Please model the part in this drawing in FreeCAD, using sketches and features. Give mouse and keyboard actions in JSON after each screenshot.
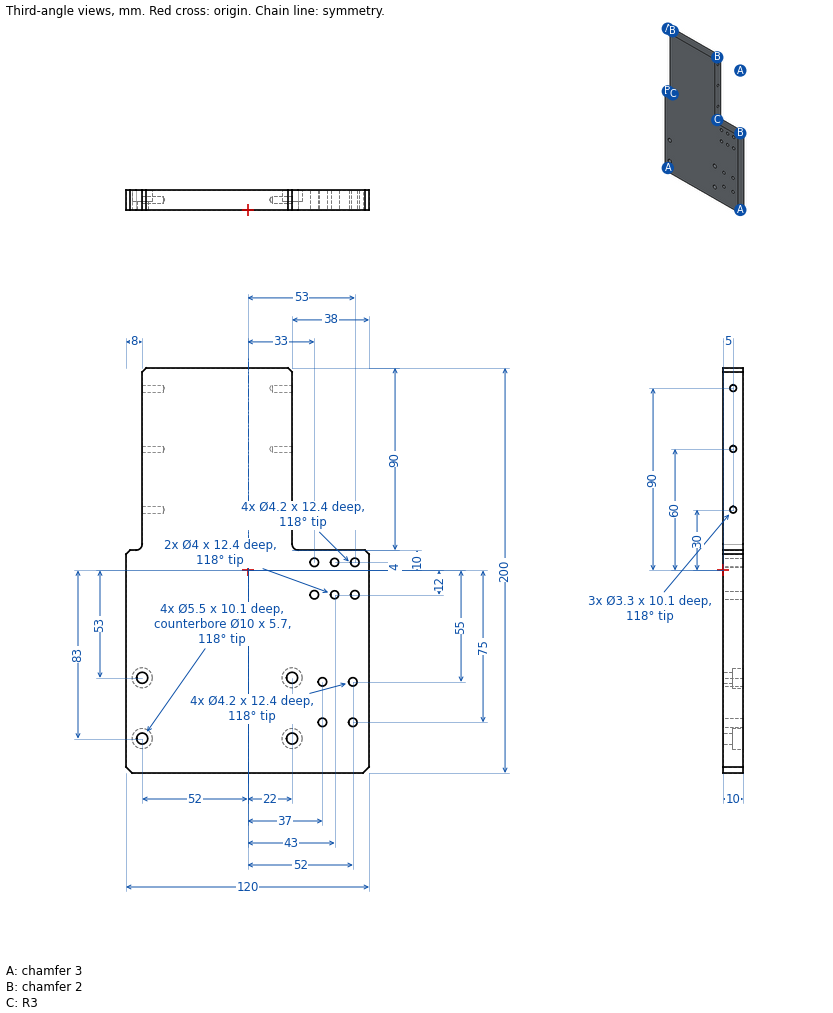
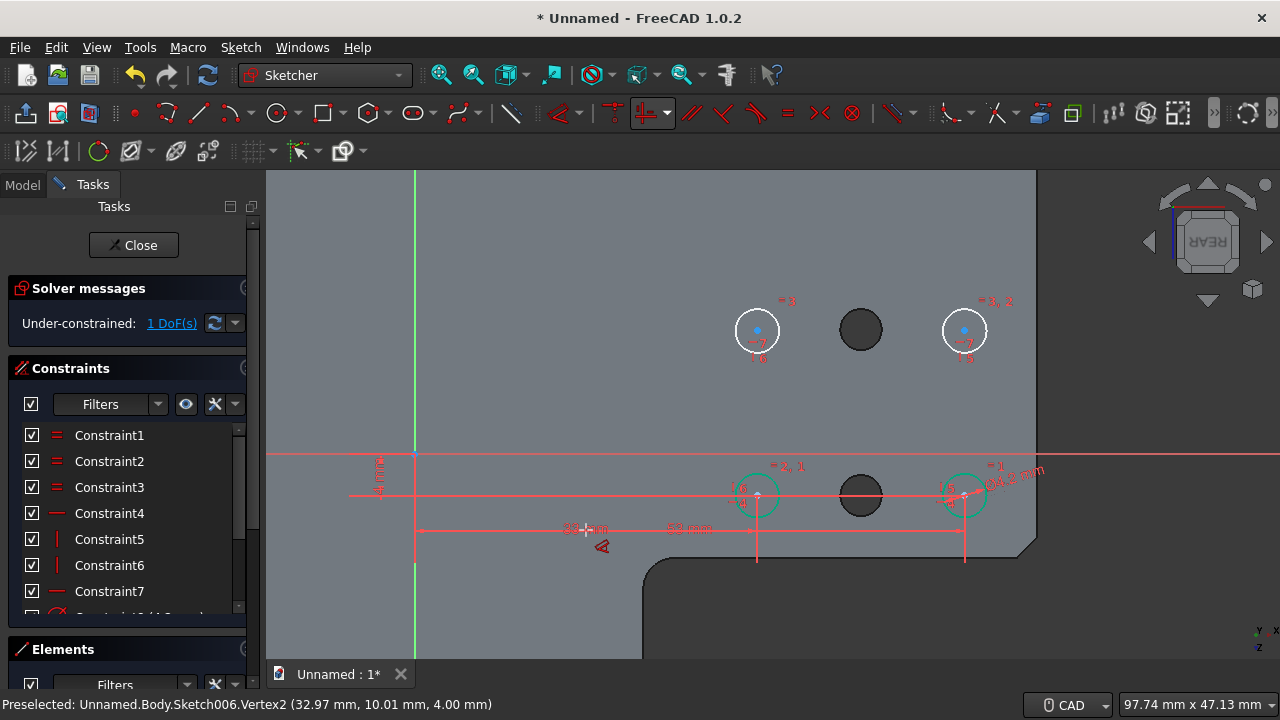
{"action": "left_click", "coordinate": [965, 331]}
{"action": "left_click", "coordinate": [381, 393]}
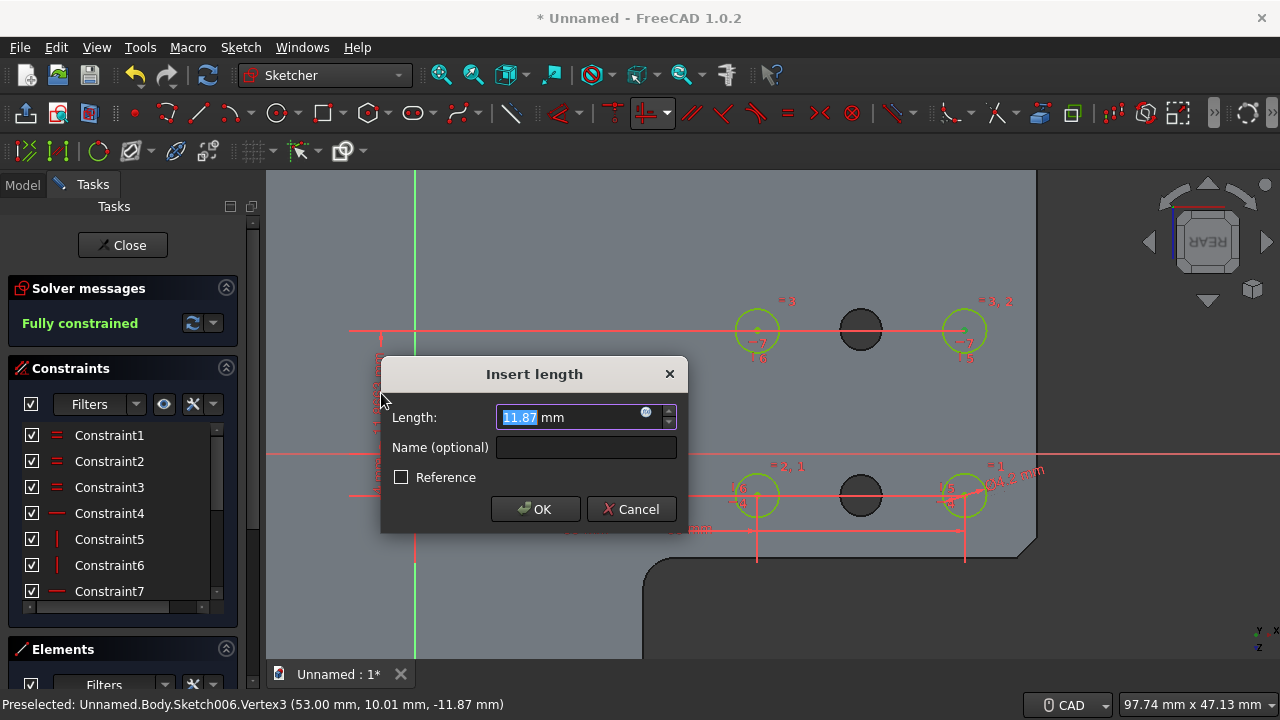
{"action": "type", "text": "12"}
{"action": "key", "text": "Return"}
{"action": "key", "text": "Escape"}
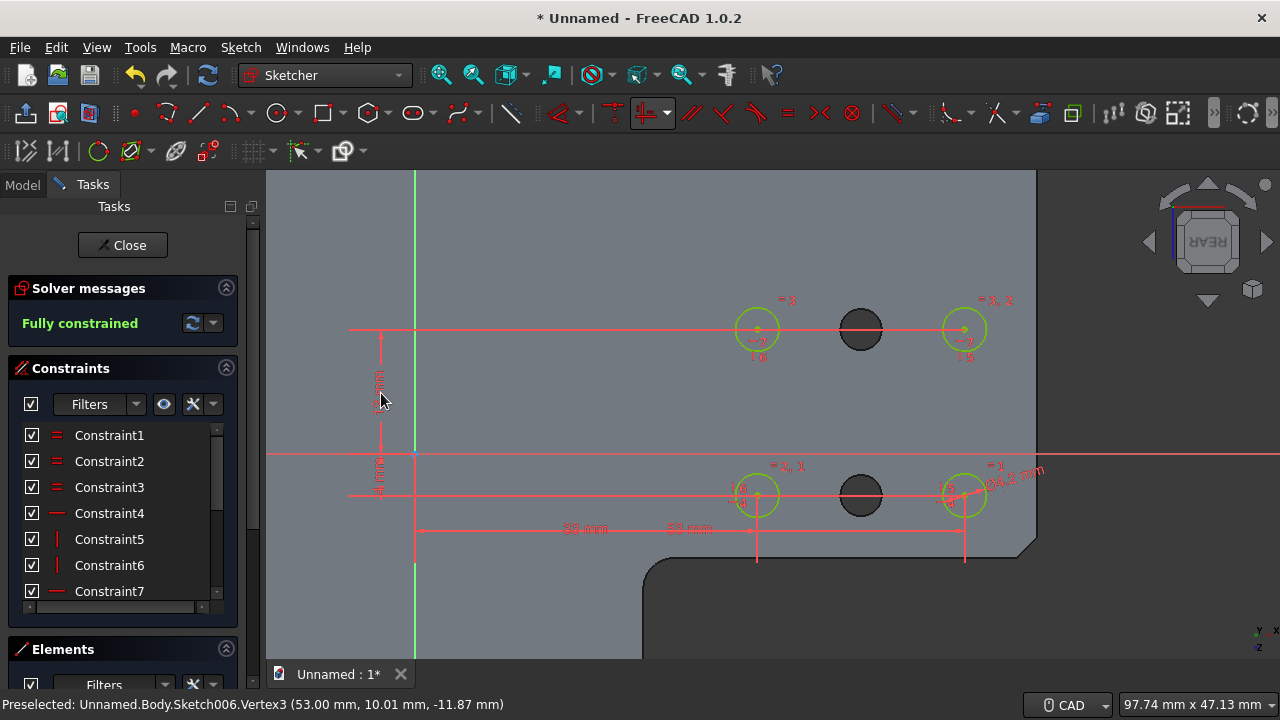
{"action": "left_click", "coordinate": [123, 245]}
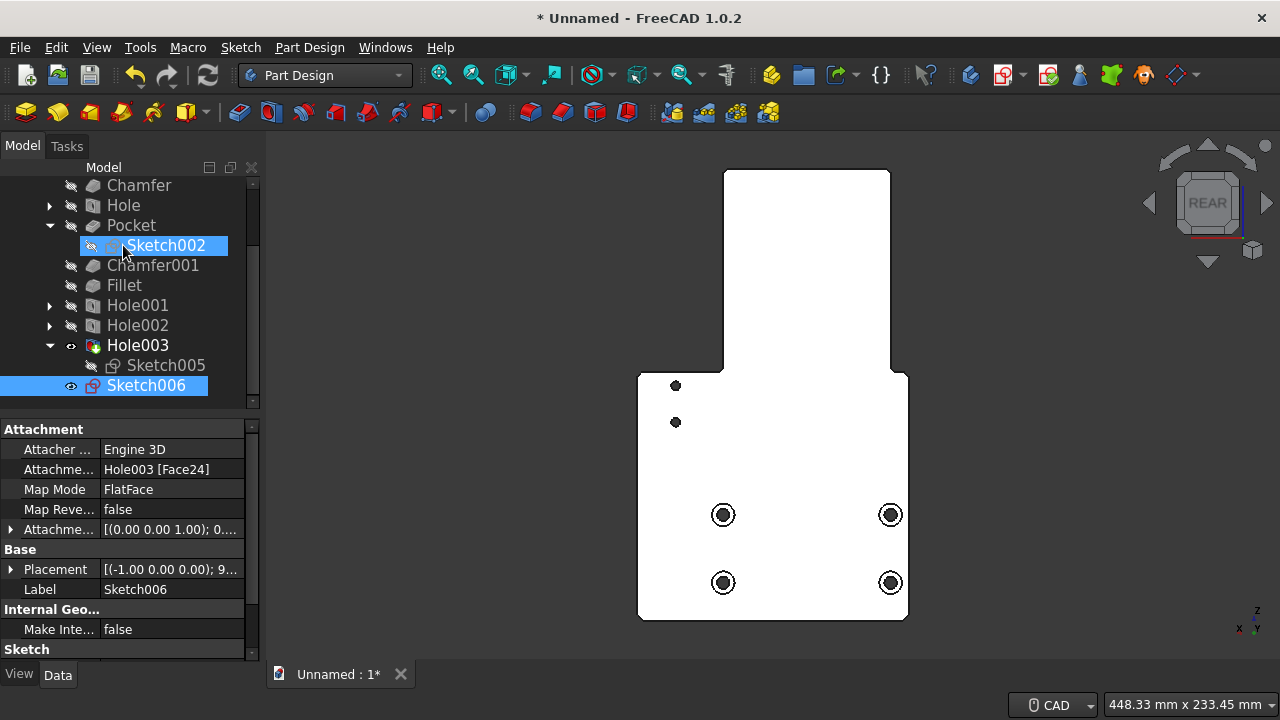
{"action": "left_click", "coordinate": [272, 112]}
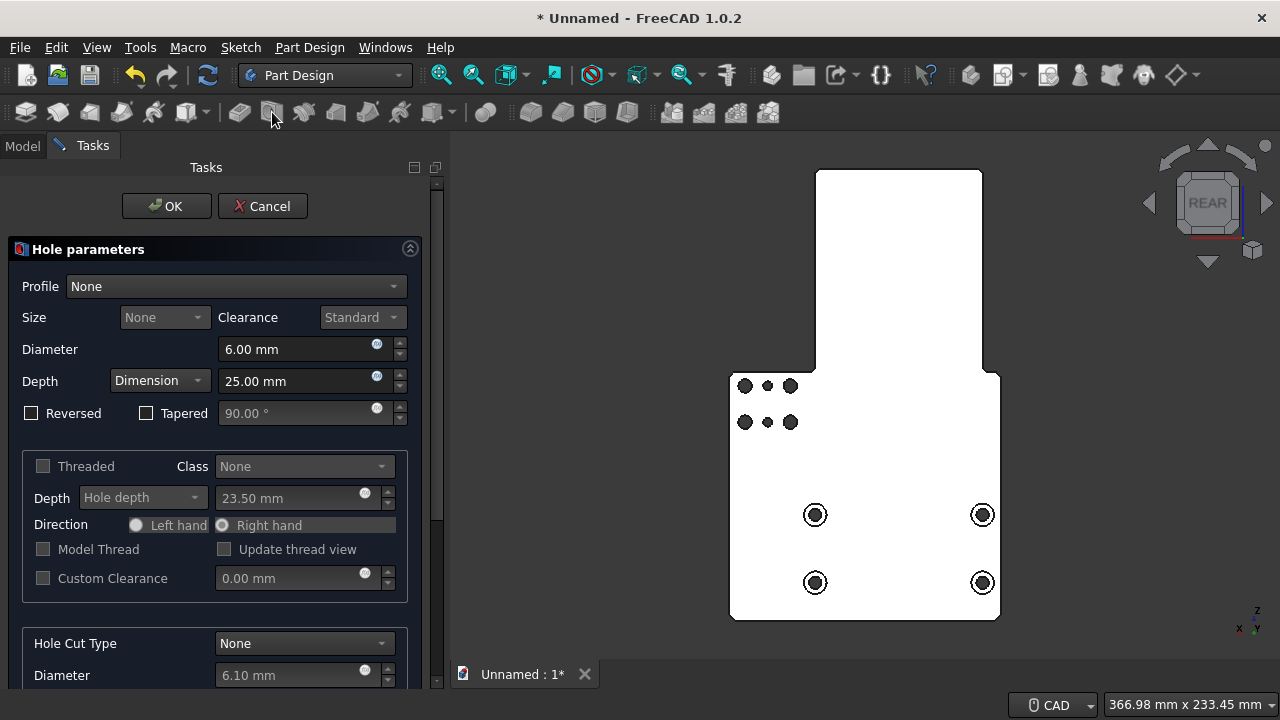
{"action": "triple_click", "coordinate": [305, 349]}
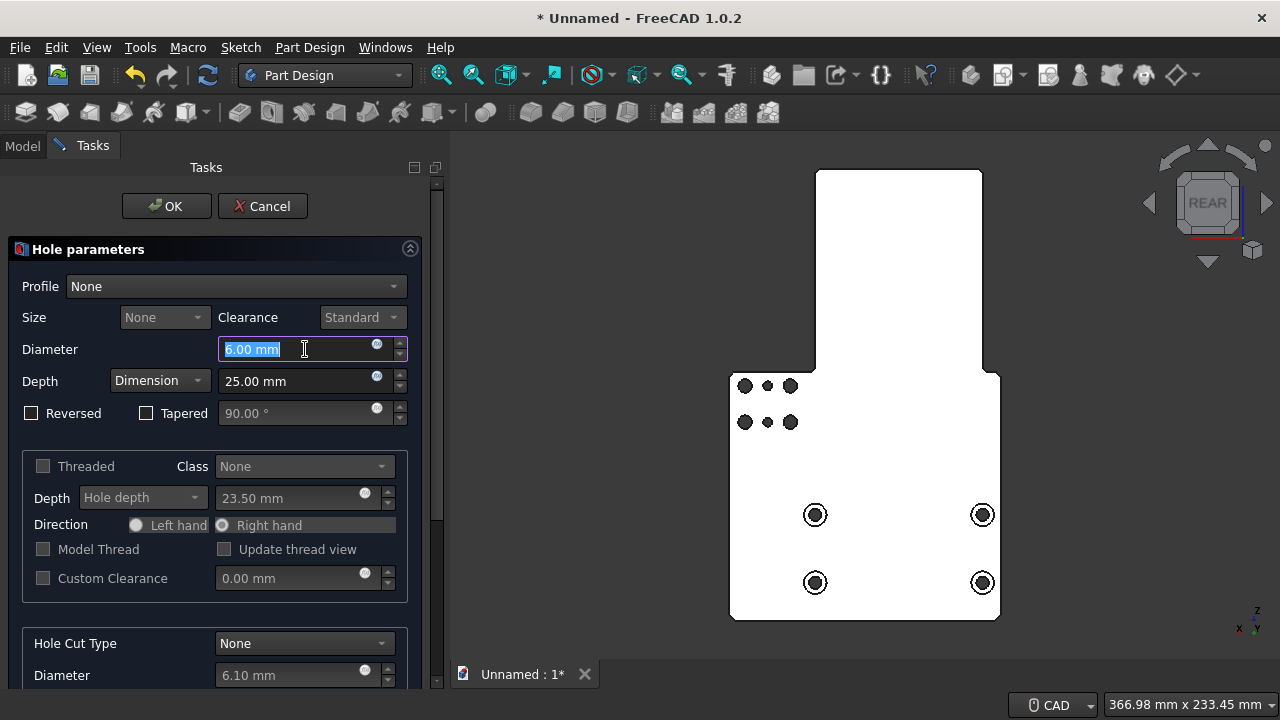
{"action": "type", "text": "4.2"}
{"action": "key", "text": "Tab"}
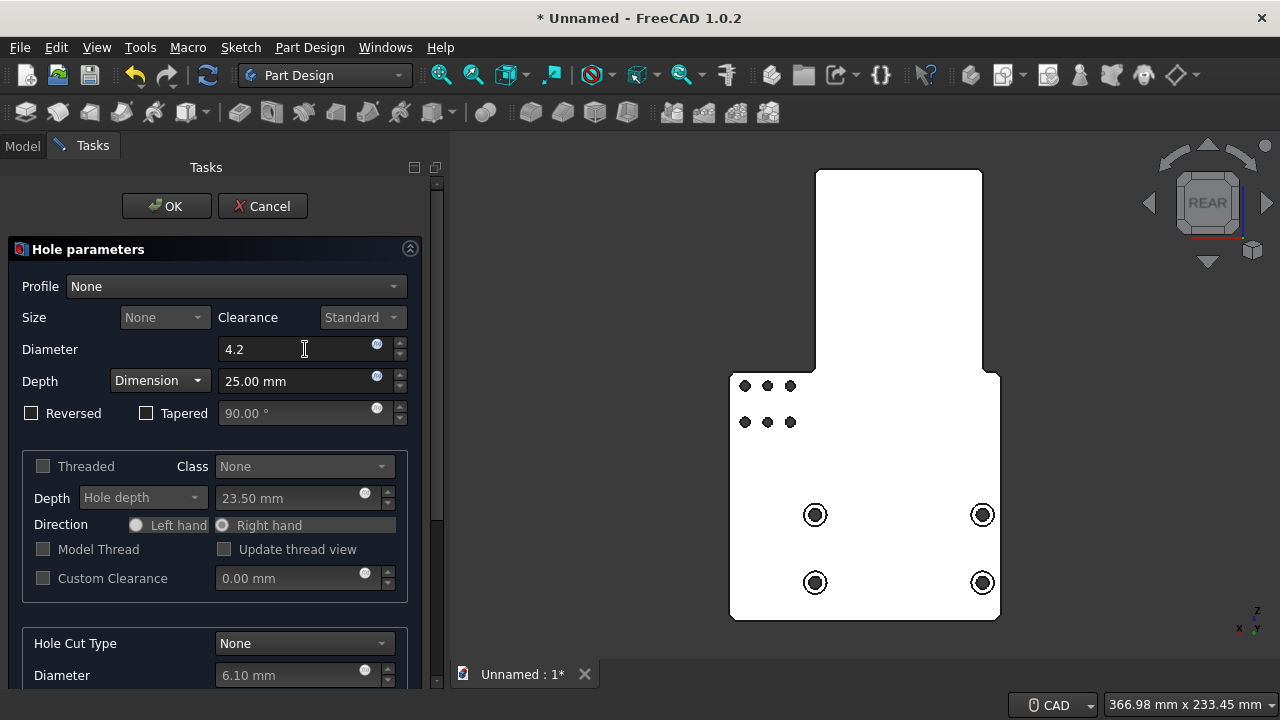
{"action": "triple_click", "coordinate": [305, 381]}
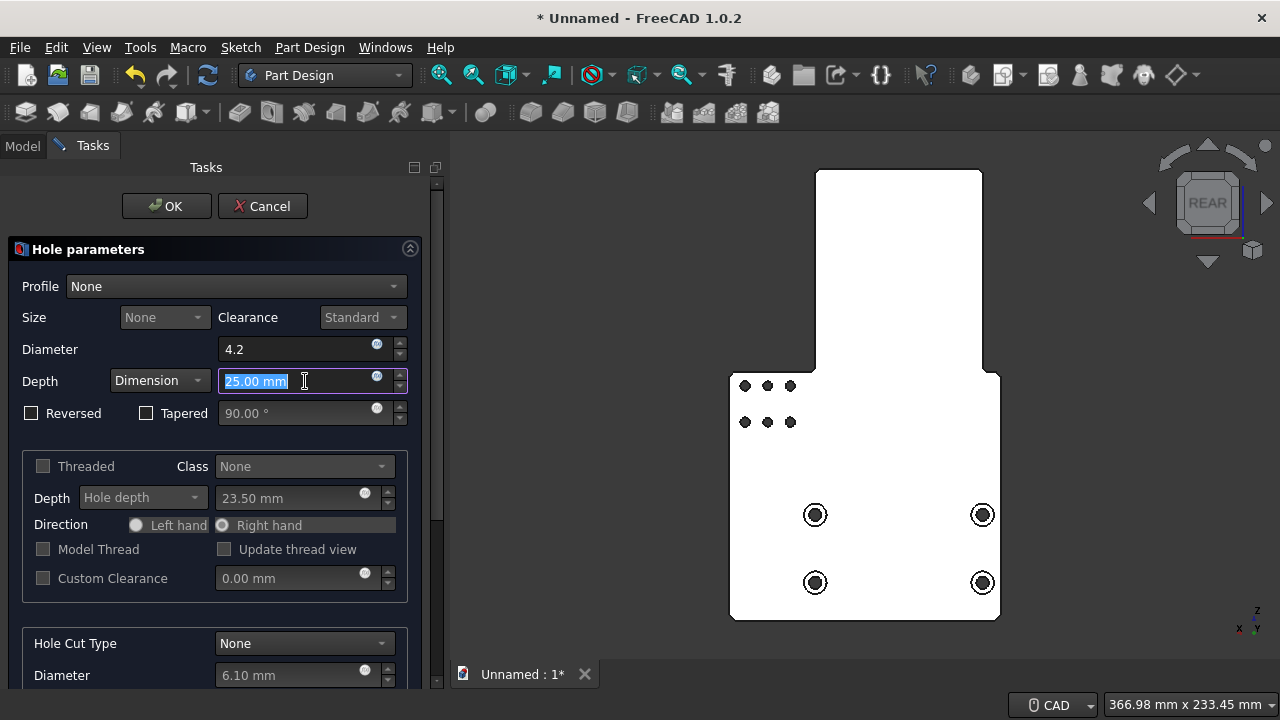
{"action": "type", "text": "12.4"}
{"action": "key", "text": "Tab"}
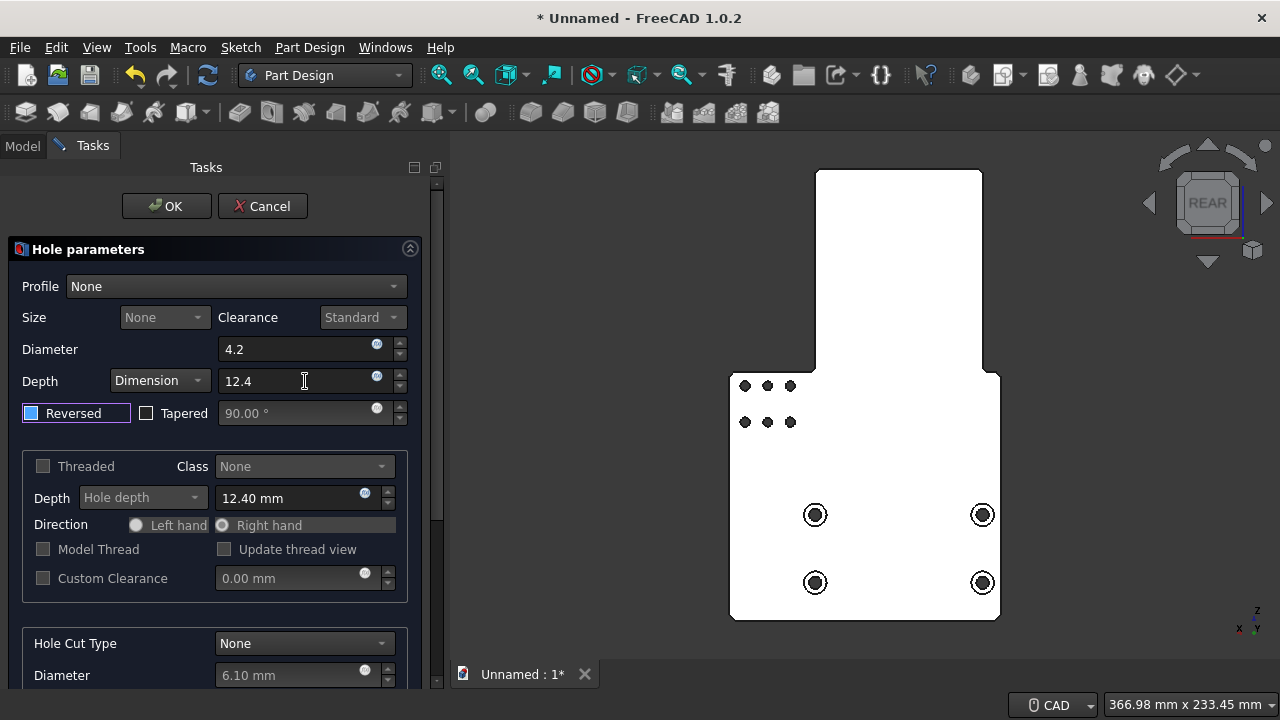
{"action": "left_click", "coordinate": [167, 206]}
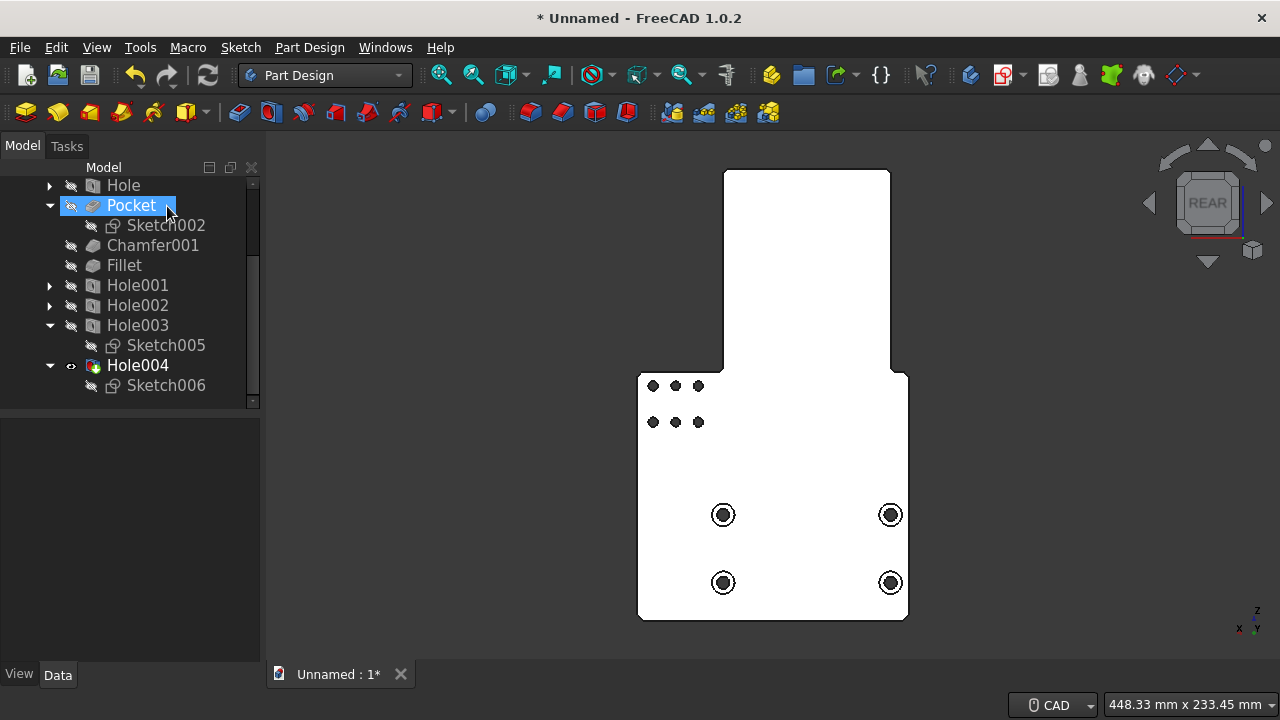
{"action": "left_click", "coordinate": [812, 459]}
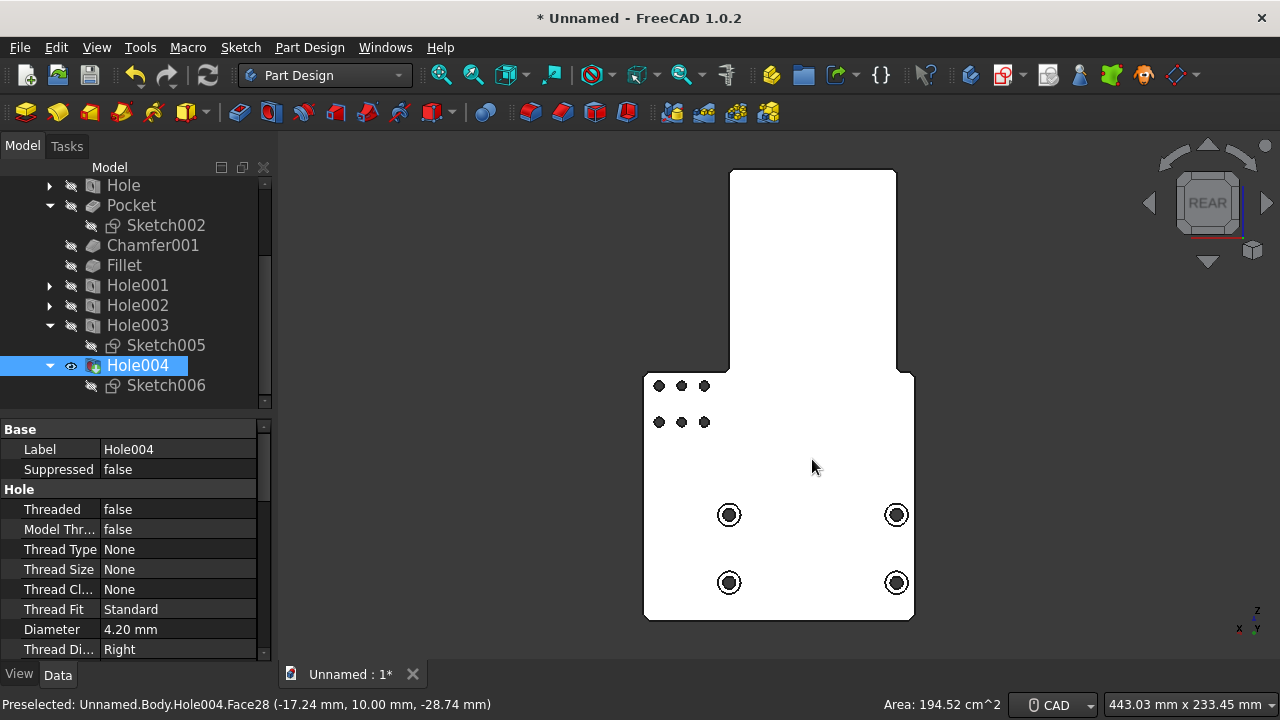
{"action": "left_click", "coordinate": [1004, 76]}